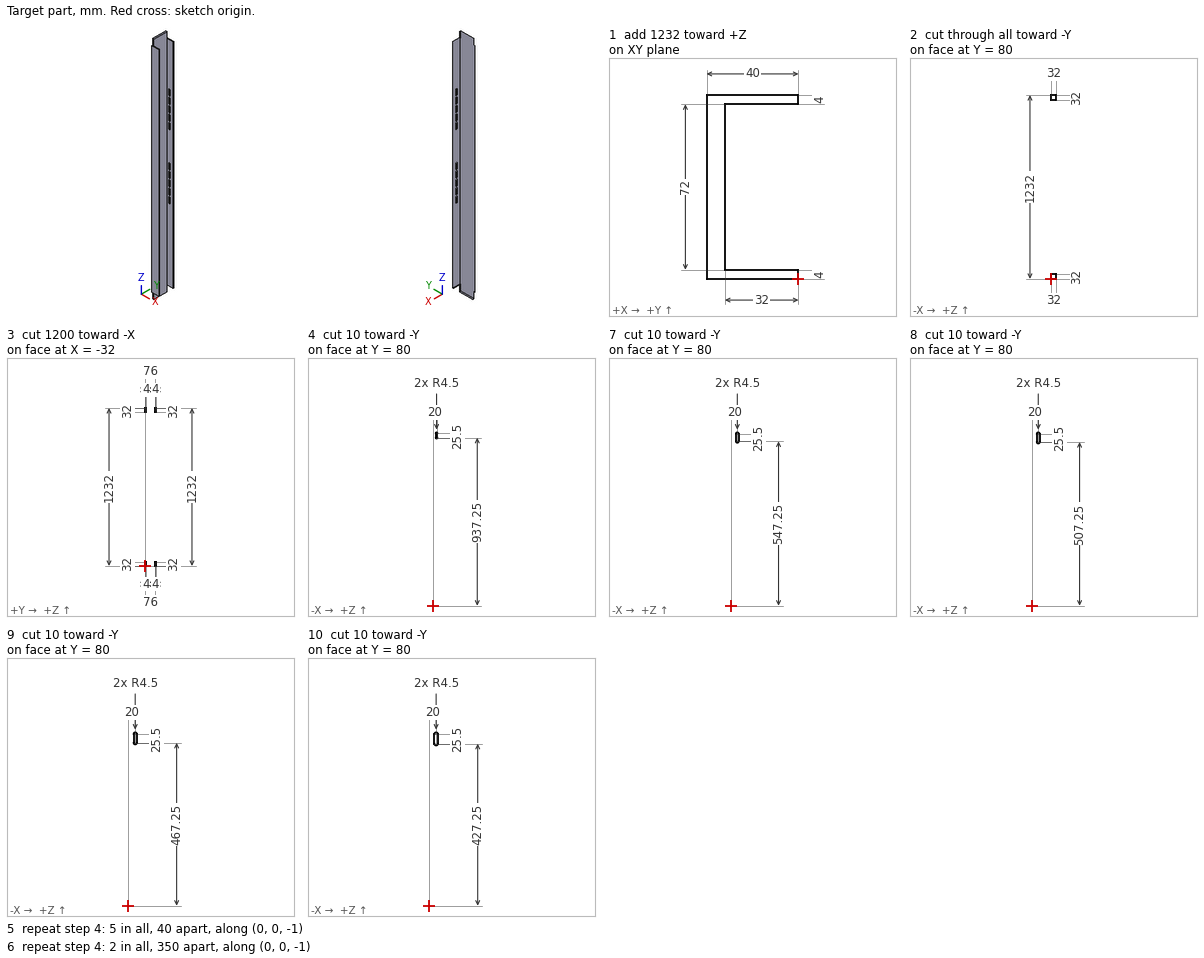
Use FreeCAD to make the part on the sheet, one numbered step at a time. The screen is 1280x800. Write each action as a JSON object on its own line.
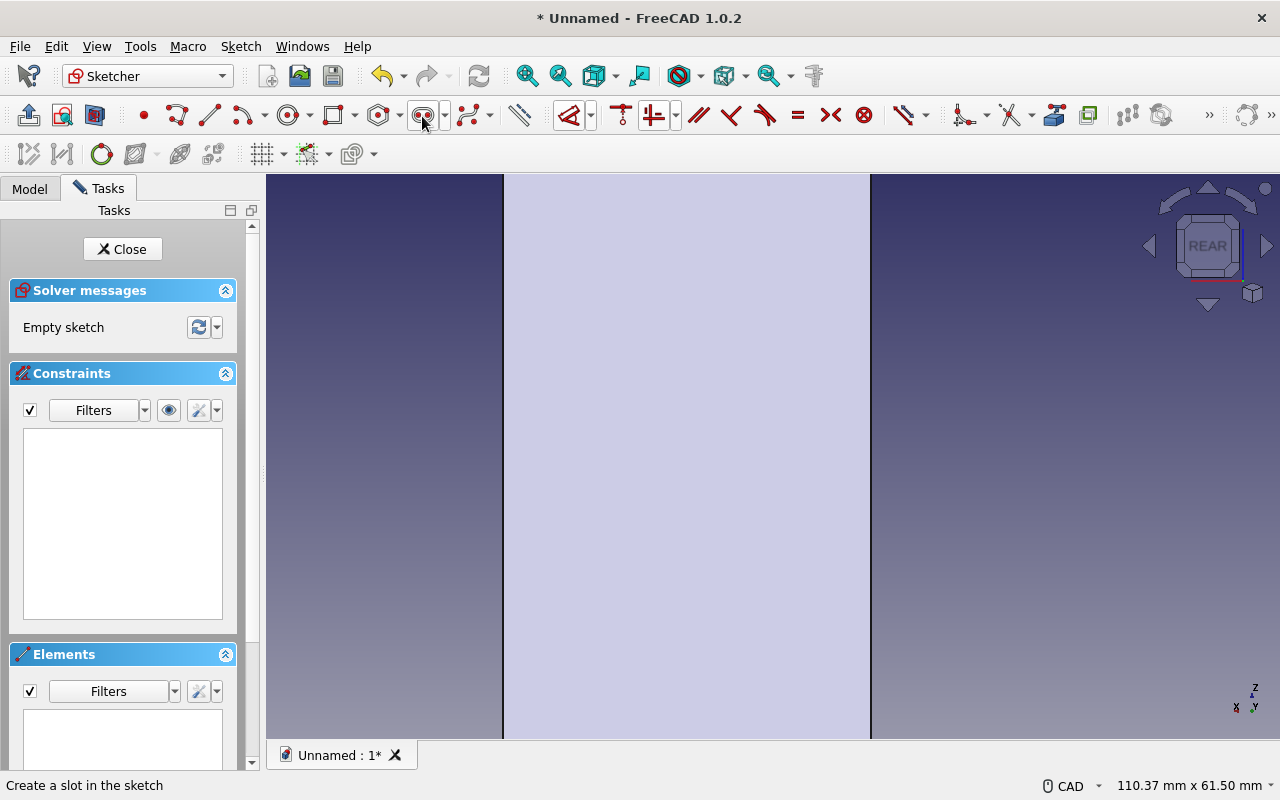
{"action": "left_click", "coordinate": [687, 564]}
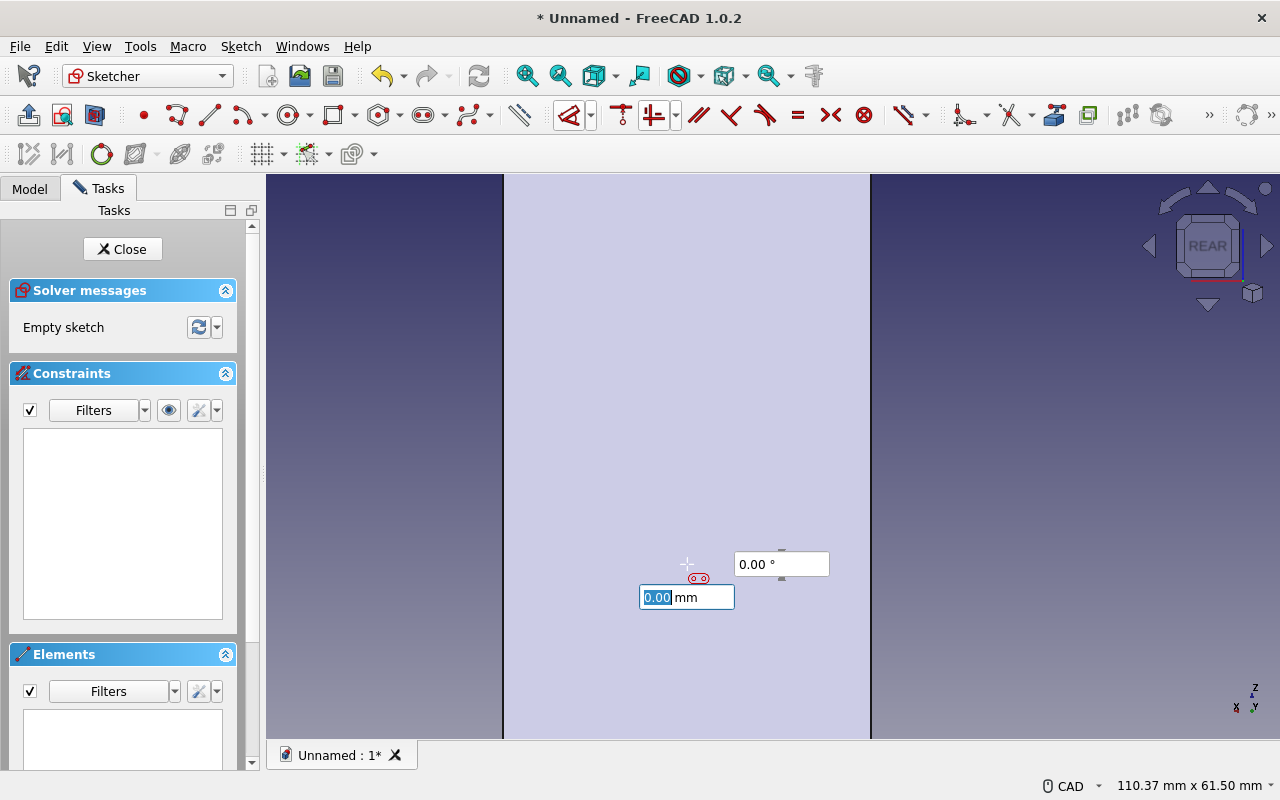
{"action": "left_click", "coordinate": [687, 330]}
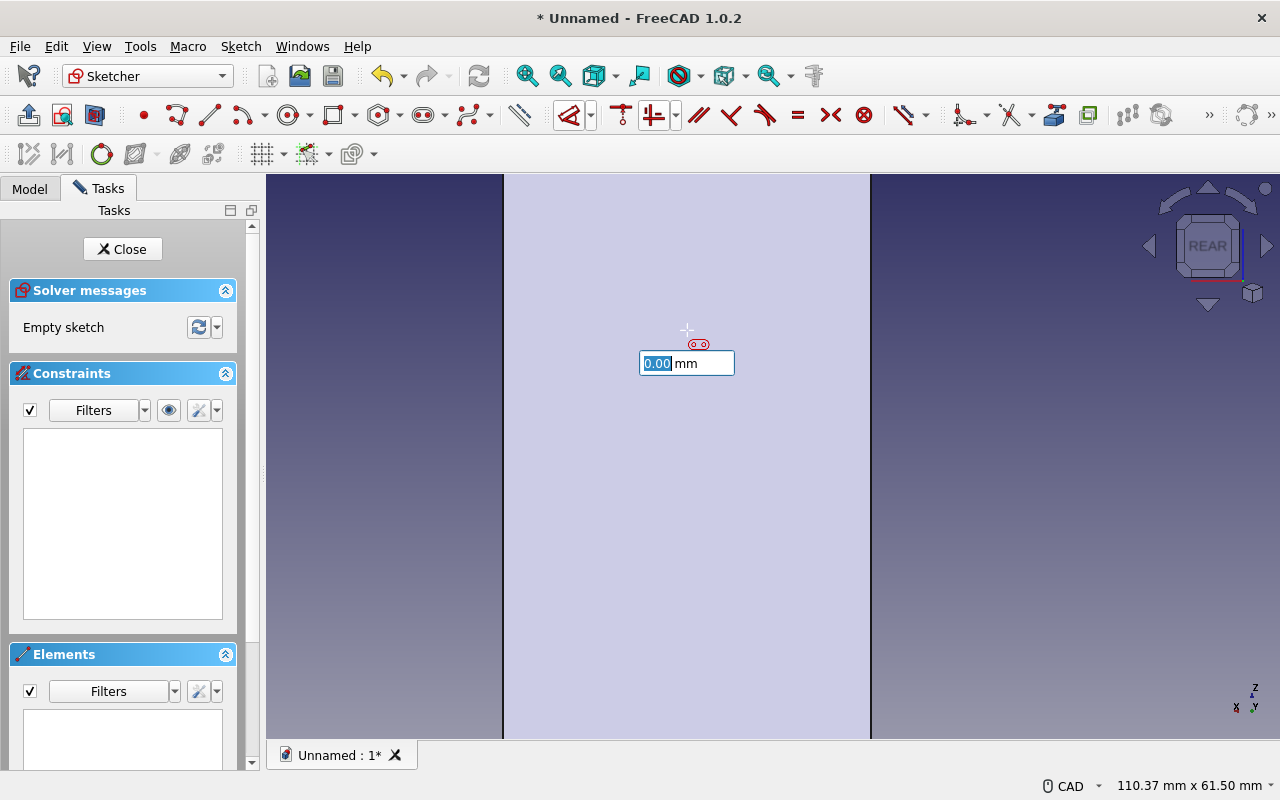
{"action": "left_click", "coordinate": [728, 447]}
{"action": "key", "text": "Escape"}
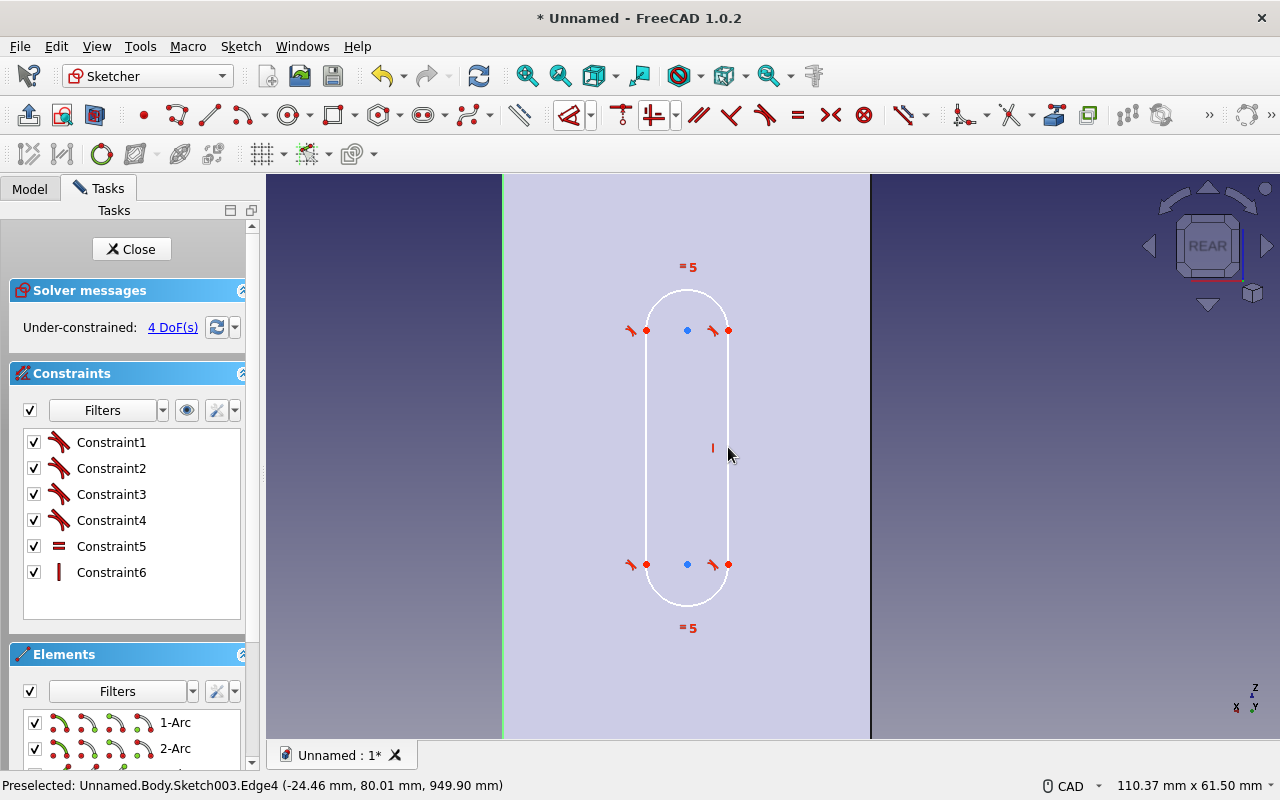
{"action": "left_click", "coordinate": [663, 598]}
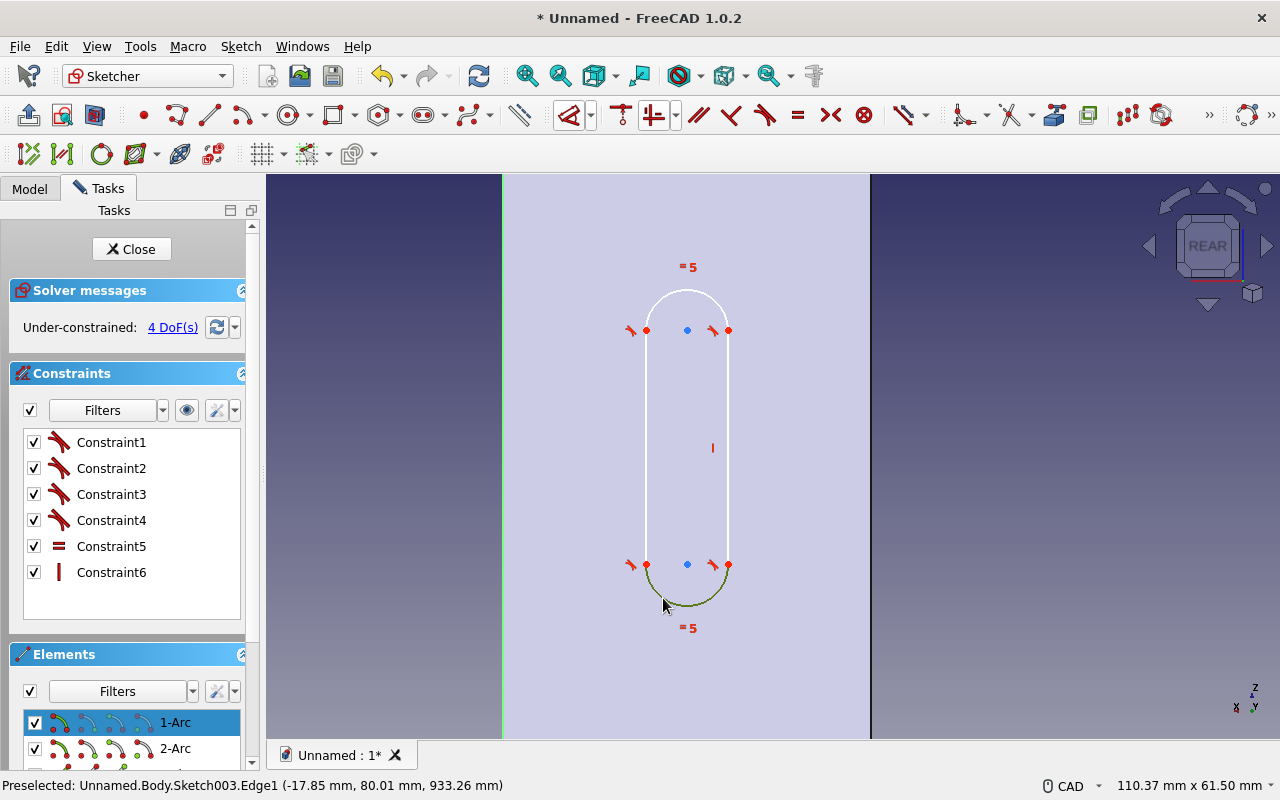
{"action": "left_click", "coordinate": [590, 116]}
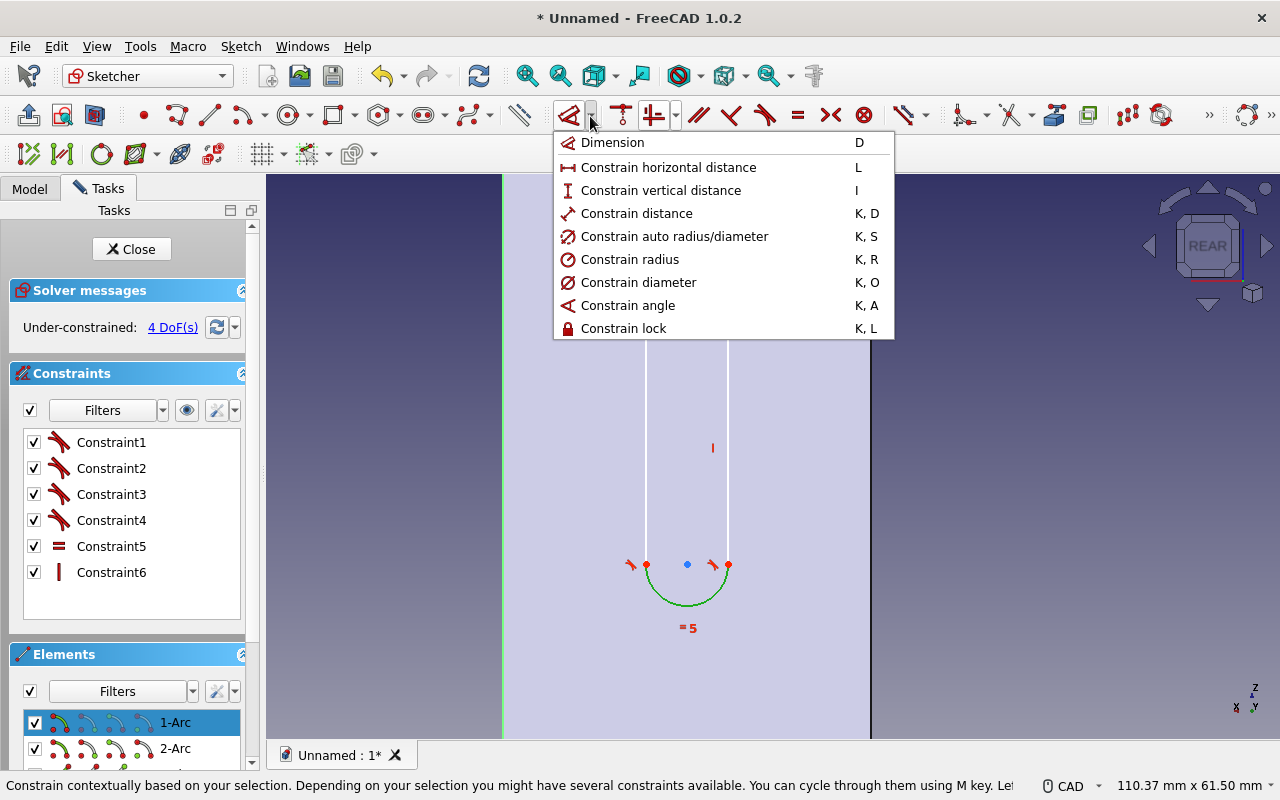
{"action": "left_click", "coordinate": [724, 260]}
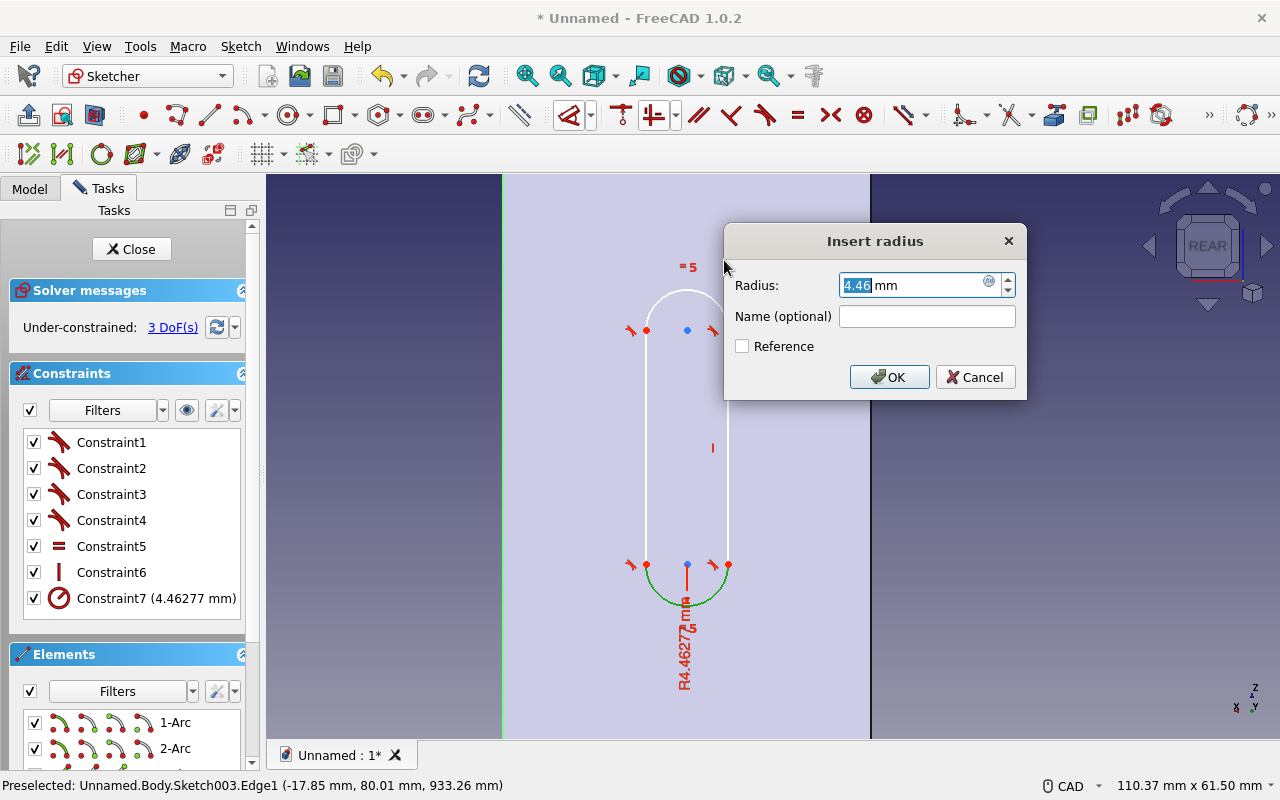
{"action": "type", "text": "4.5"}
{"action": "key", "text": "Return"}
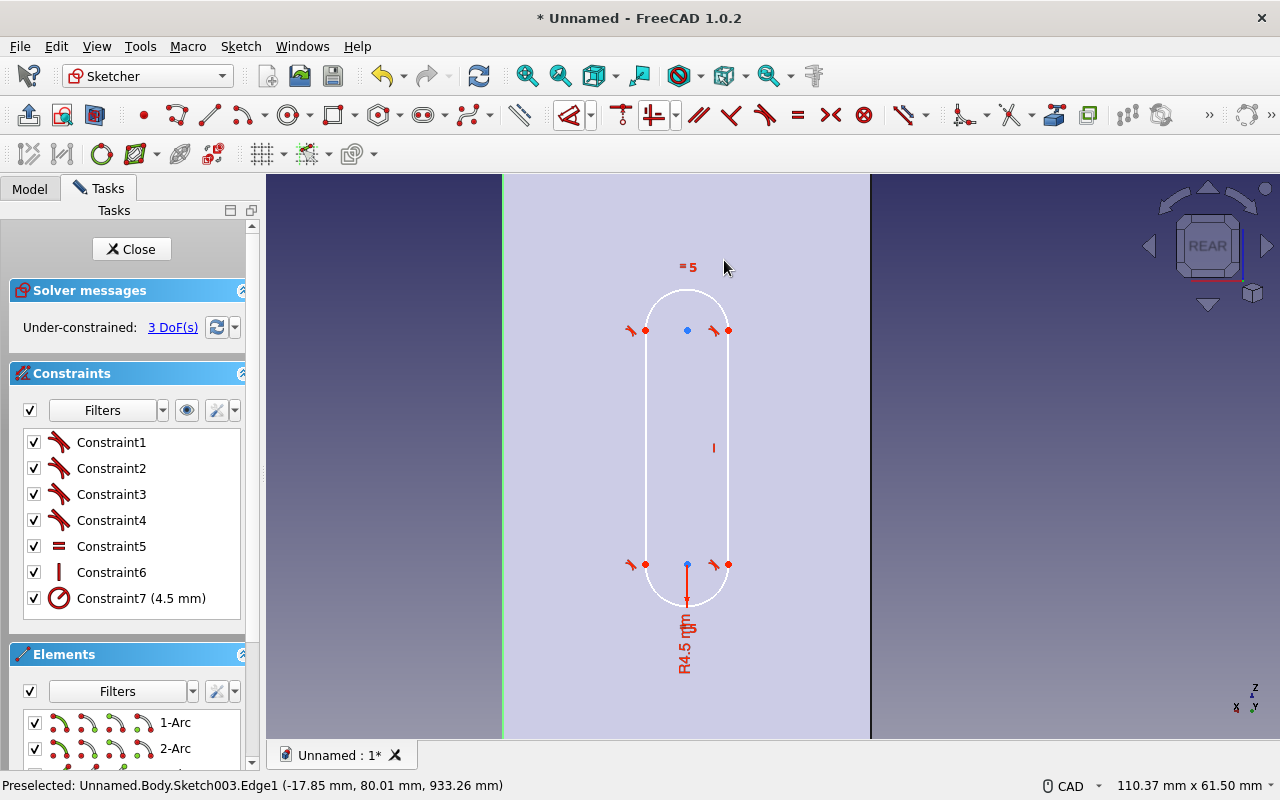
{"action": "left_click", "coordinate": [687, 565]}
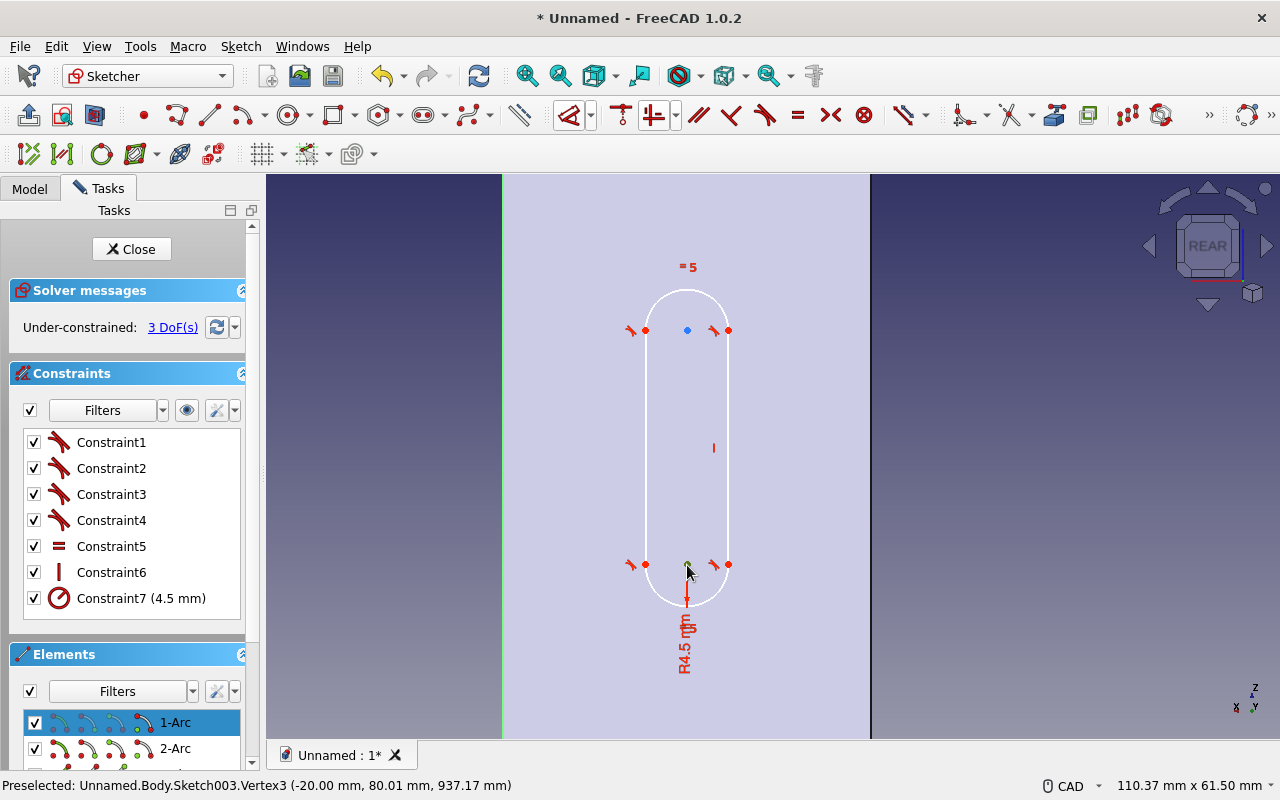
{"action": "left_click", "coordinate": [590, 116]}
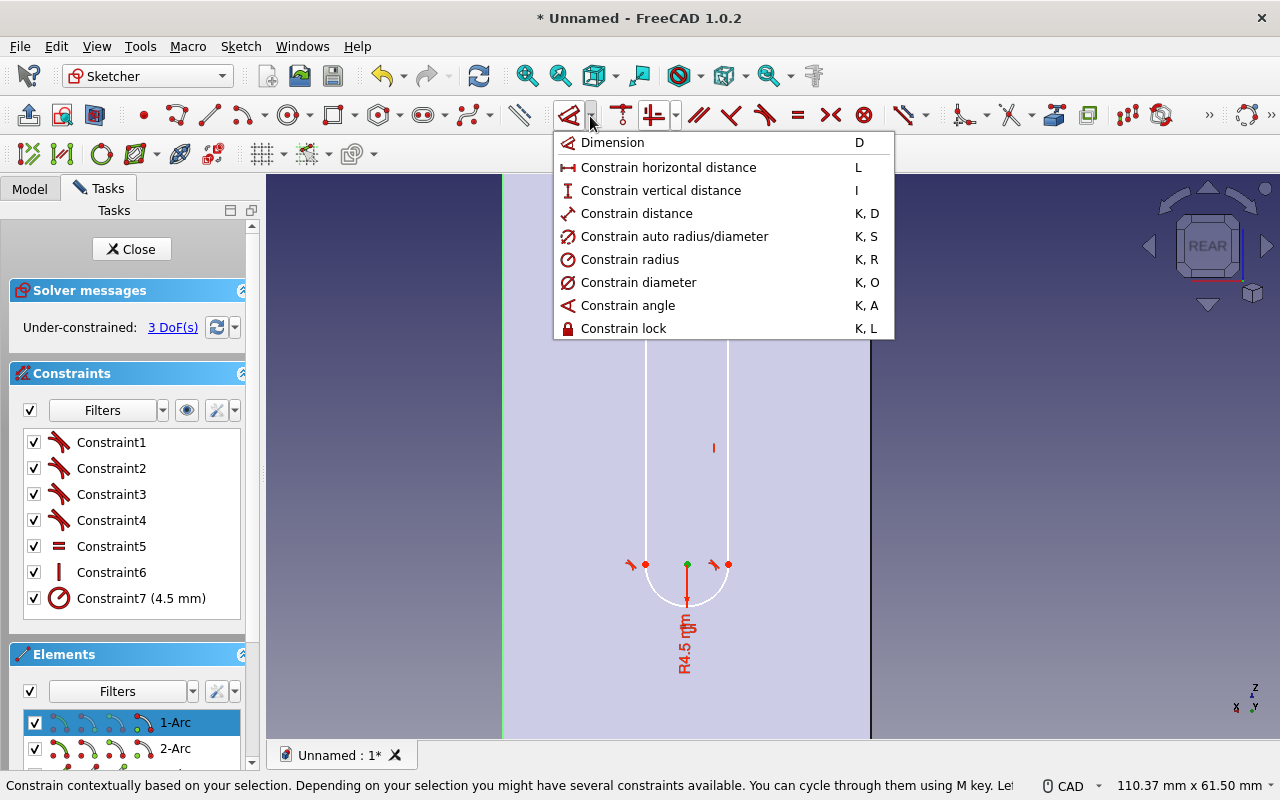
{"action": "left_click", "coordinate": [724, 168]}